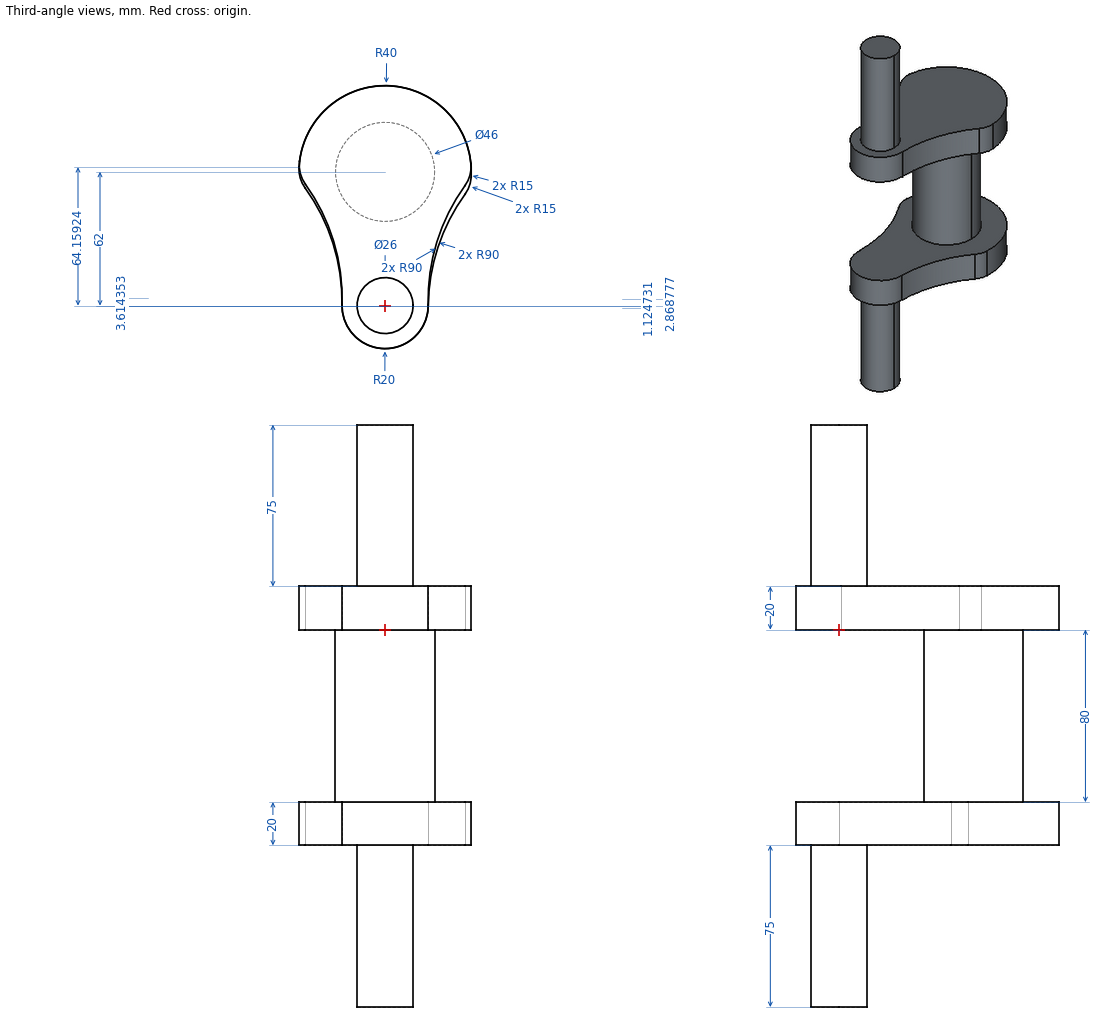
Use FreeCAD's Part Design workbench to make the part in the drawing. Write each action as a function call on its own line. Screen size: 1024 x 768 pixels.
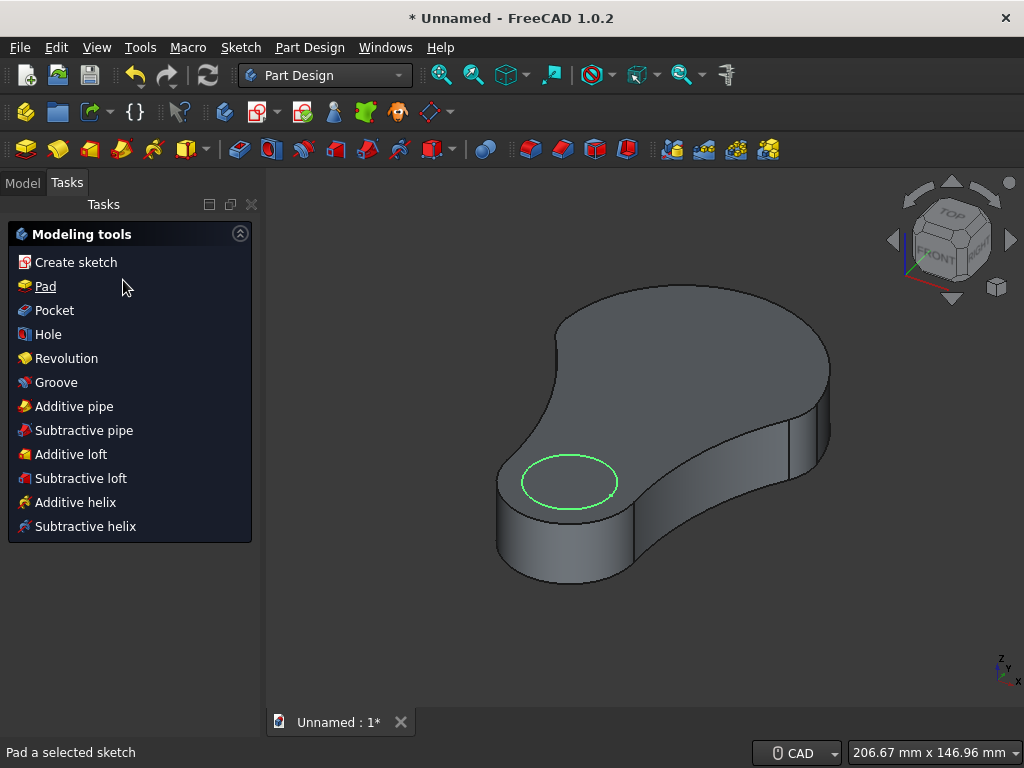
click(26, 150)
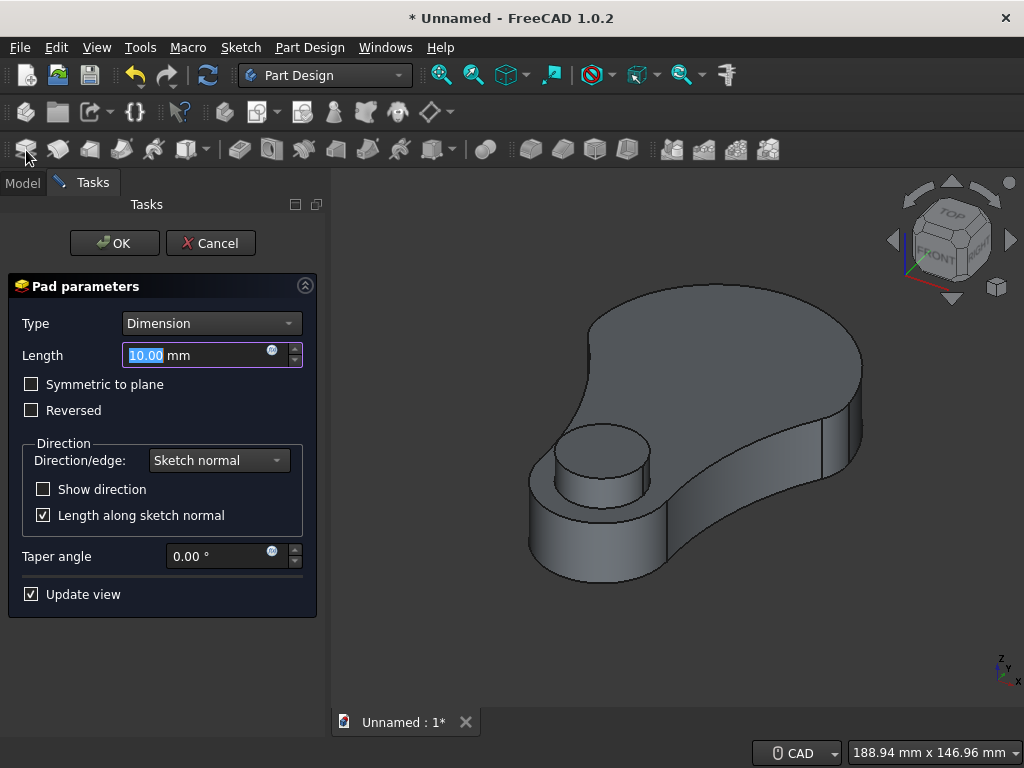
text(75)
key(Tab)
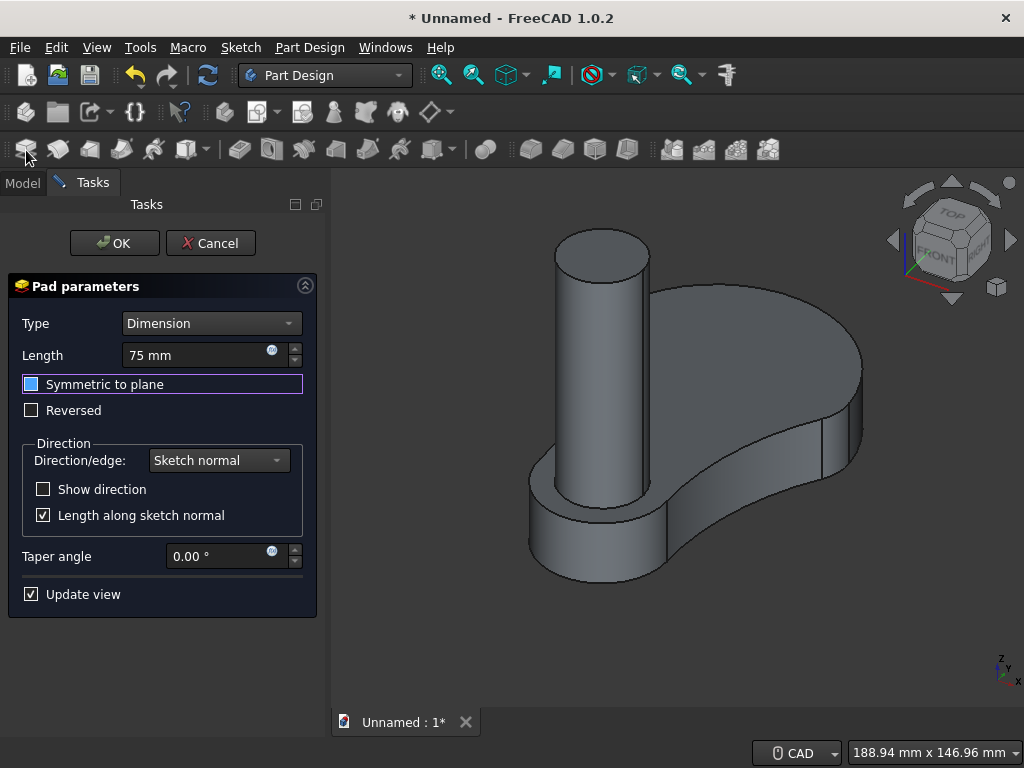
click(115, 243)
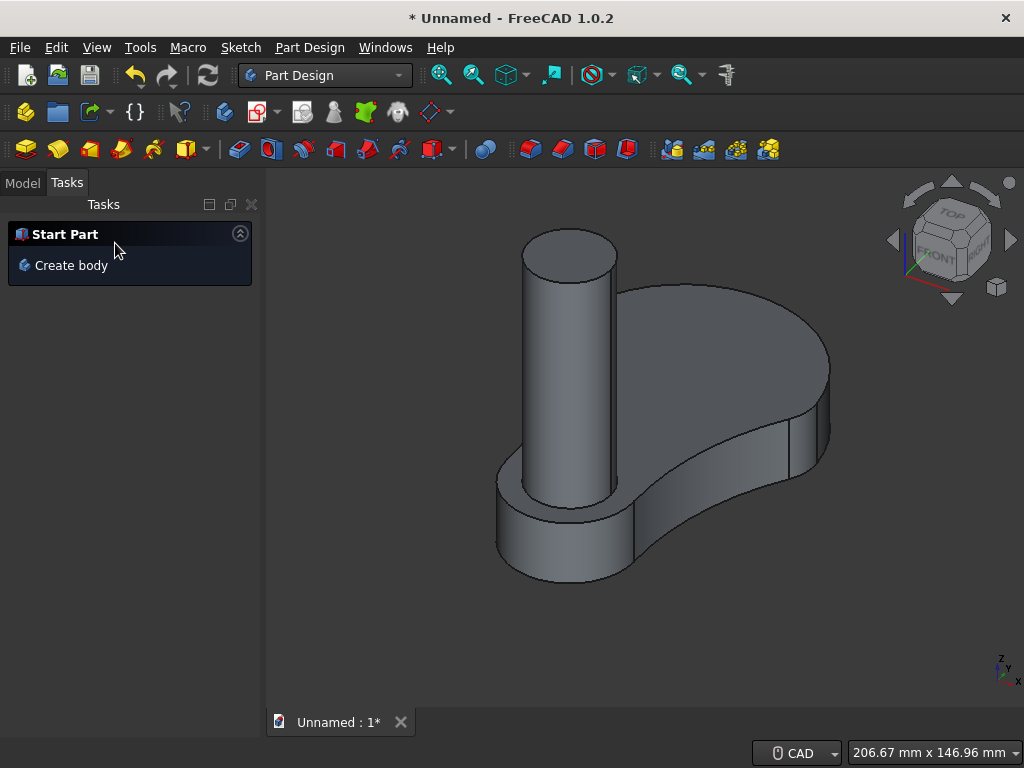
click(442, 76)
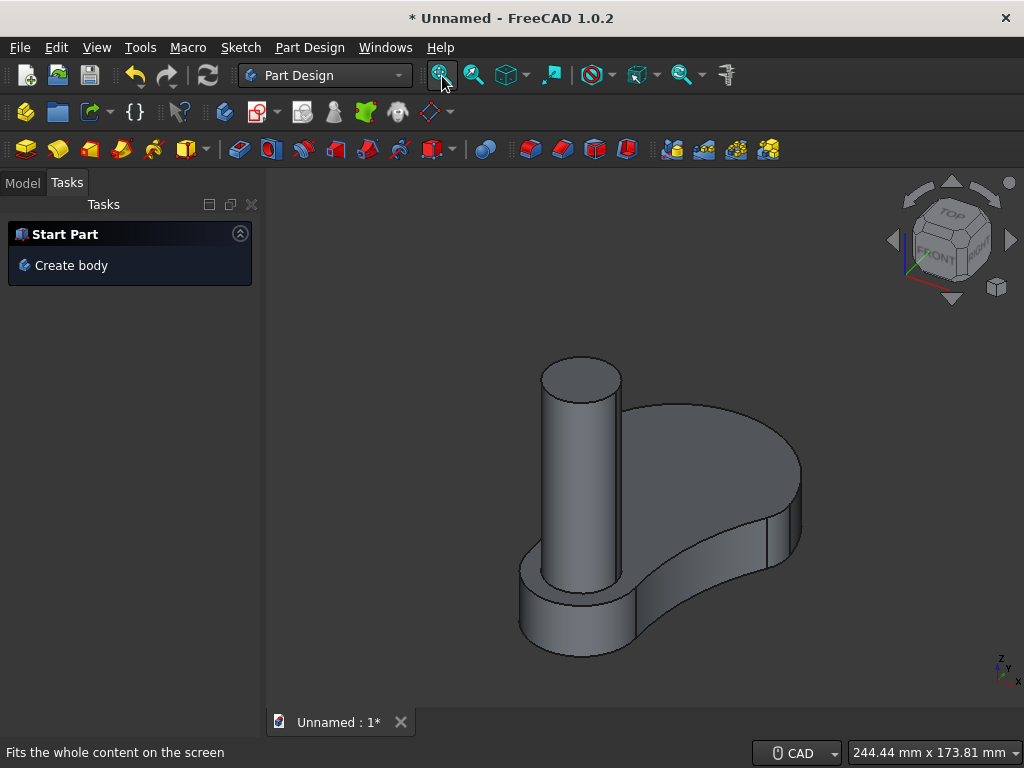
click(258, 112)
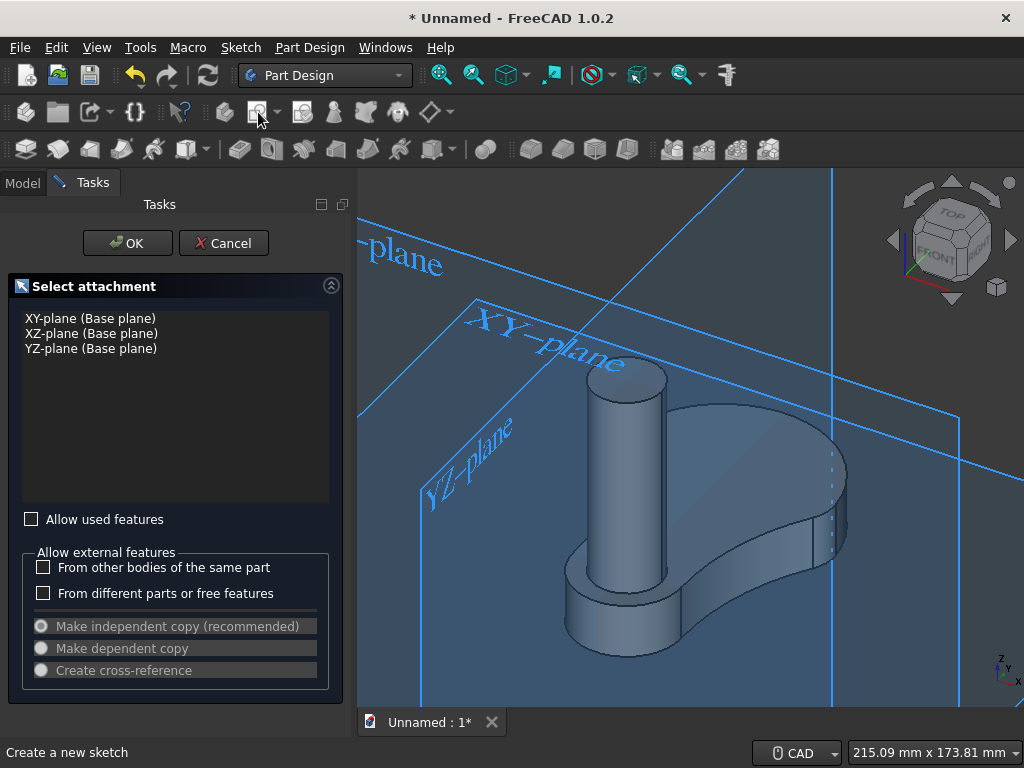
click(82, 318)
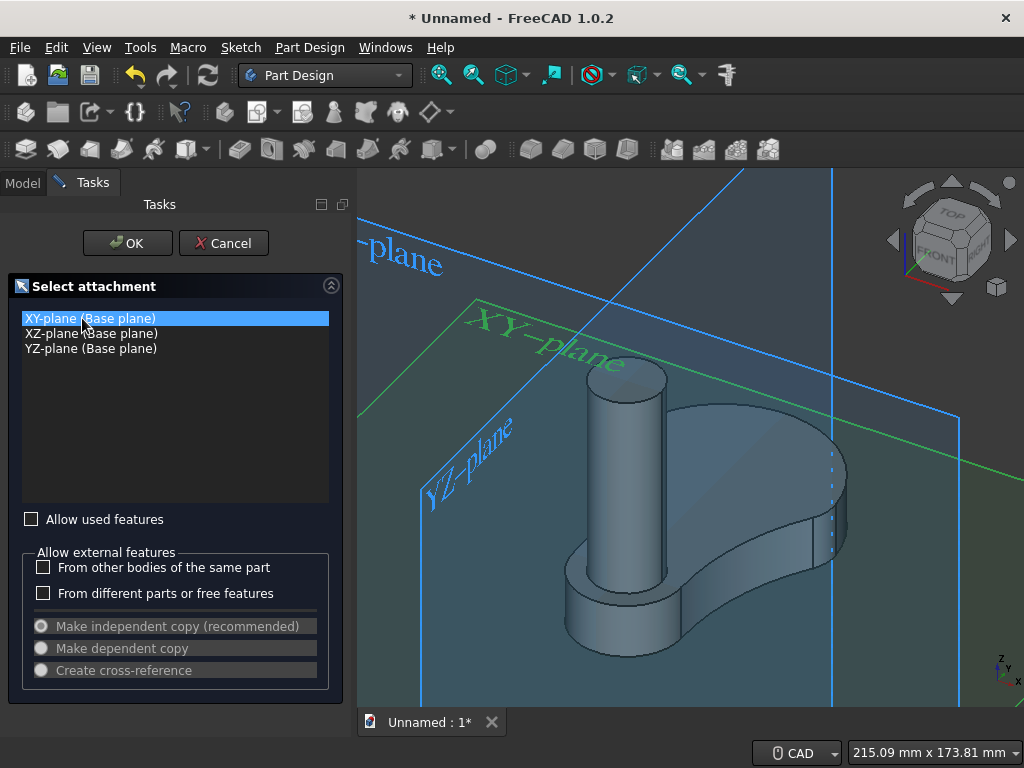
click(128, 243)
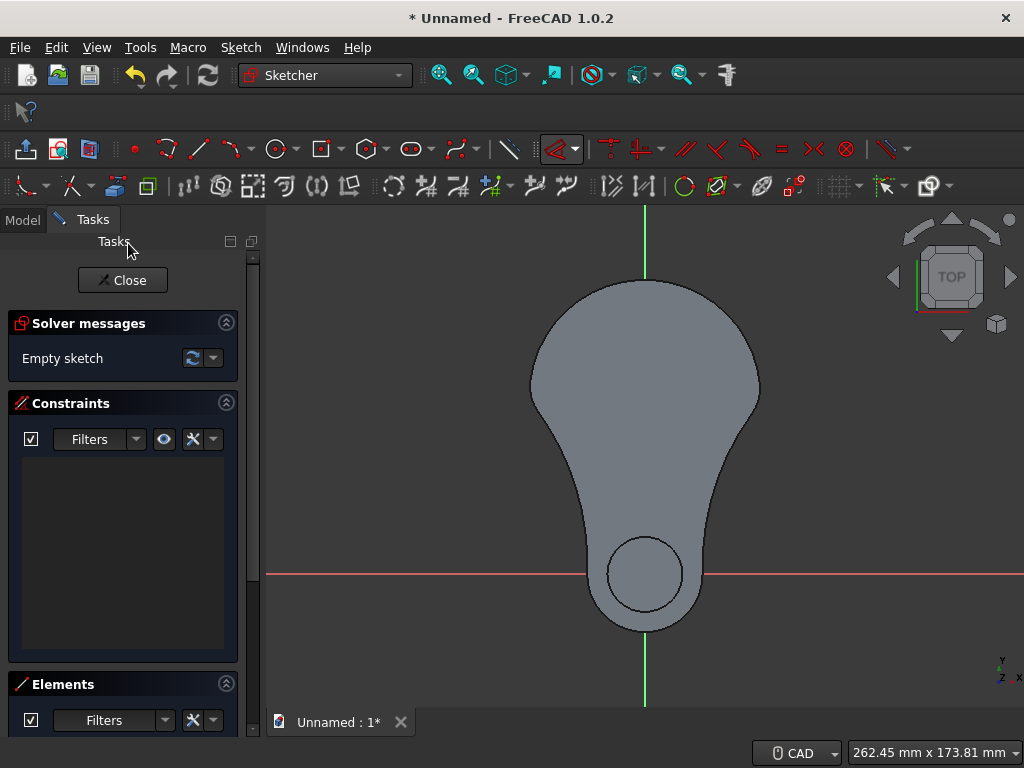
click(90, 150)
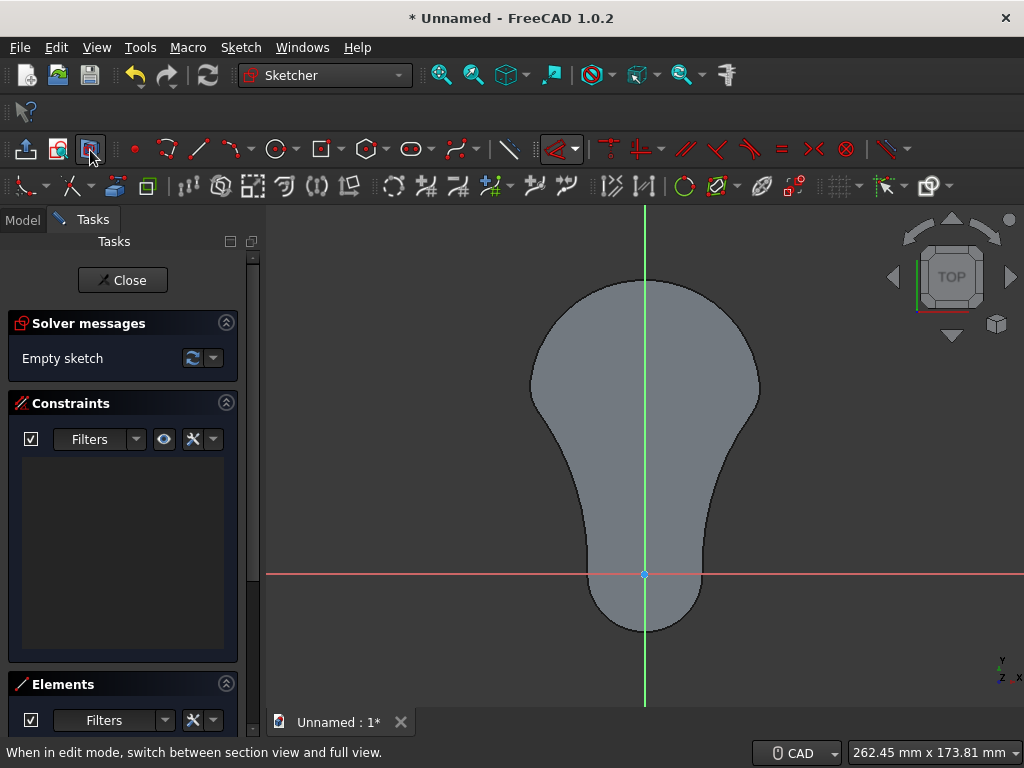
click(276, 150)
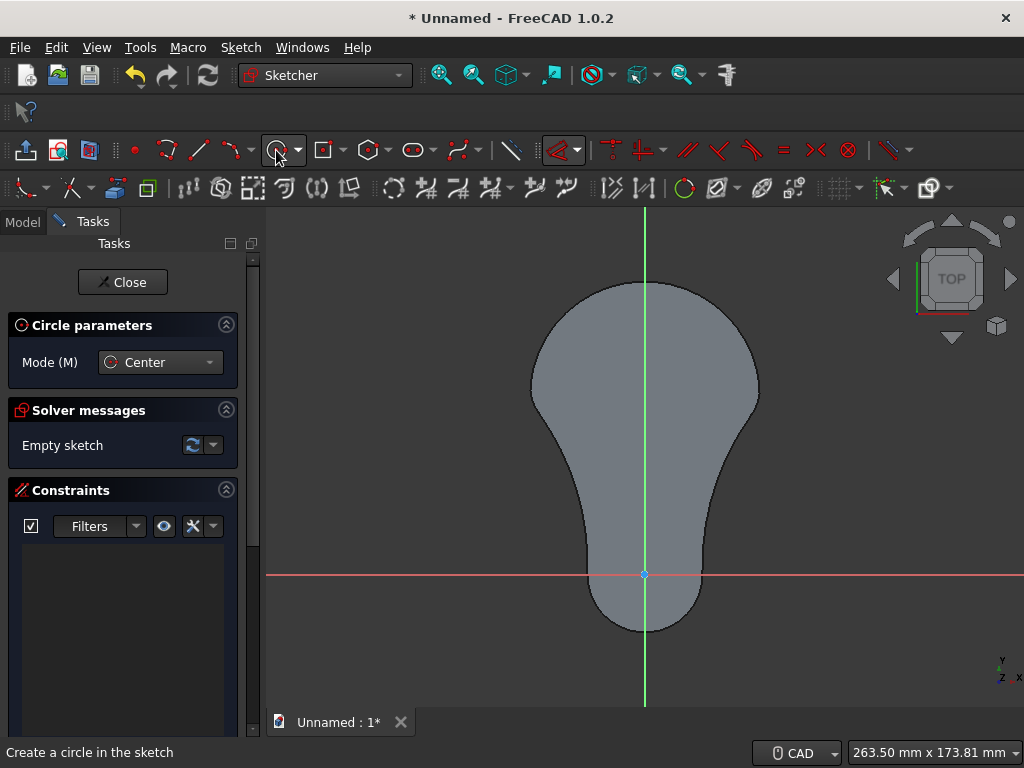
click(645, 397)
move(692, 350)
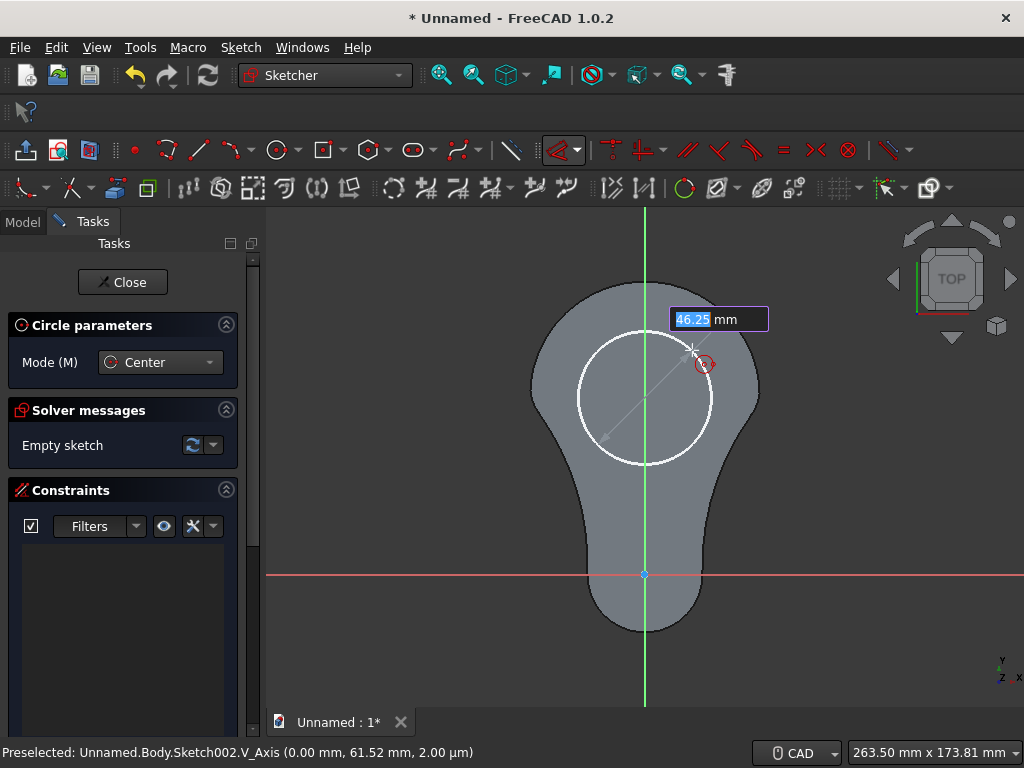
text(46)
key(Return)
key(Escape)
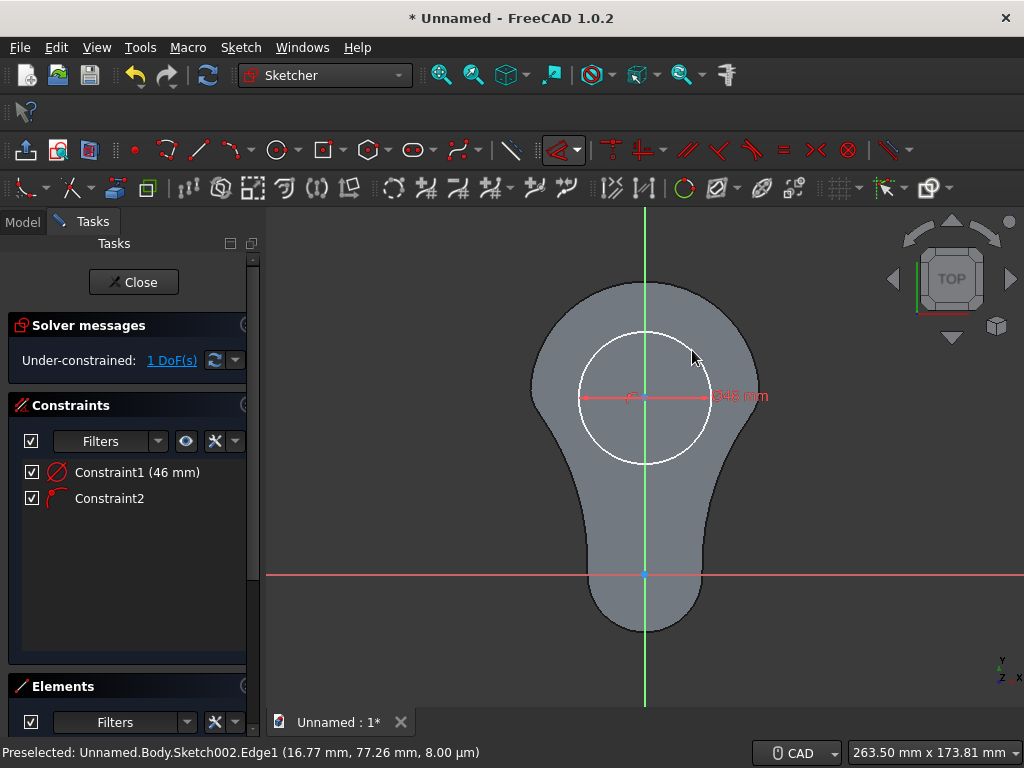
click(645, 398)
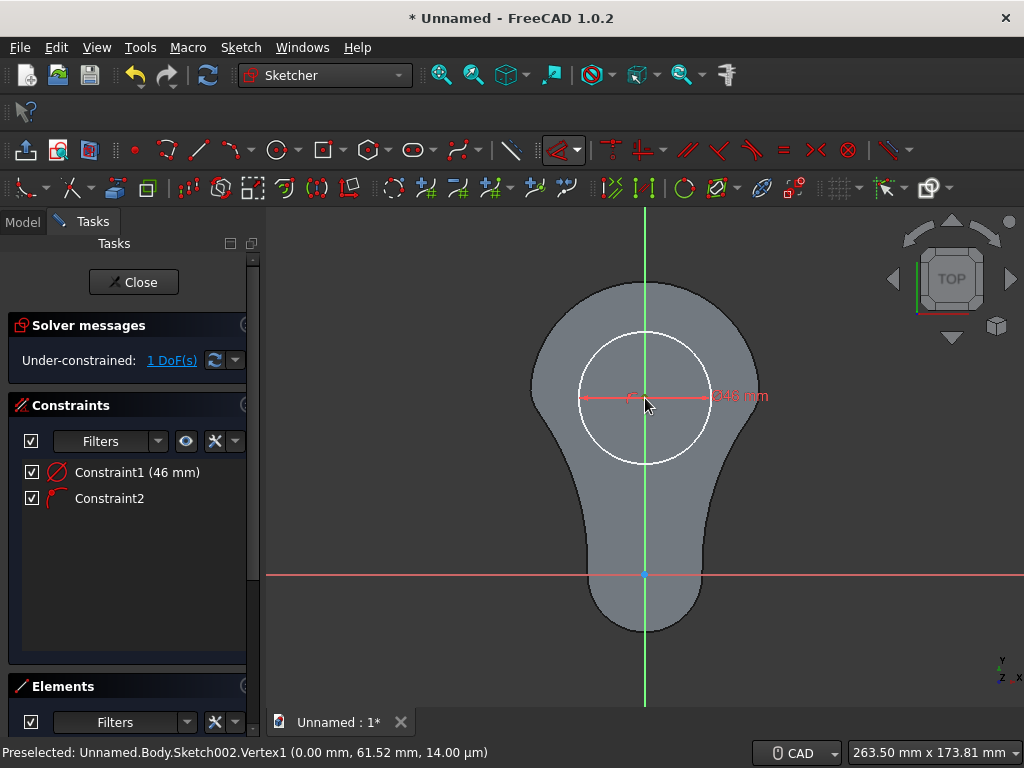
key(i)